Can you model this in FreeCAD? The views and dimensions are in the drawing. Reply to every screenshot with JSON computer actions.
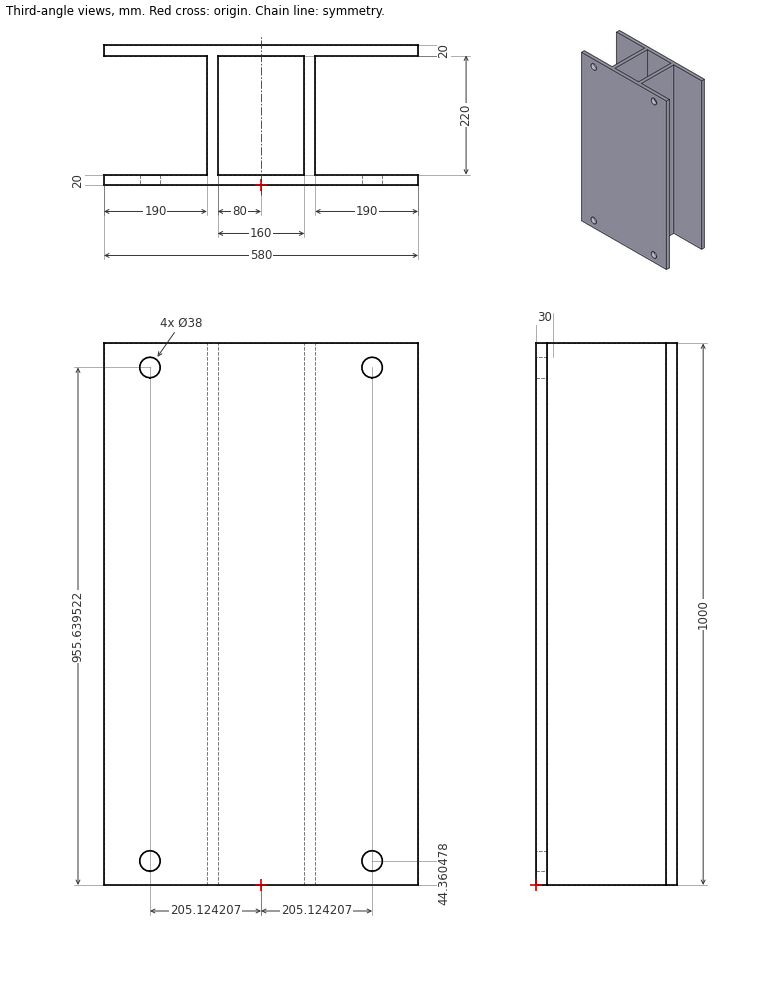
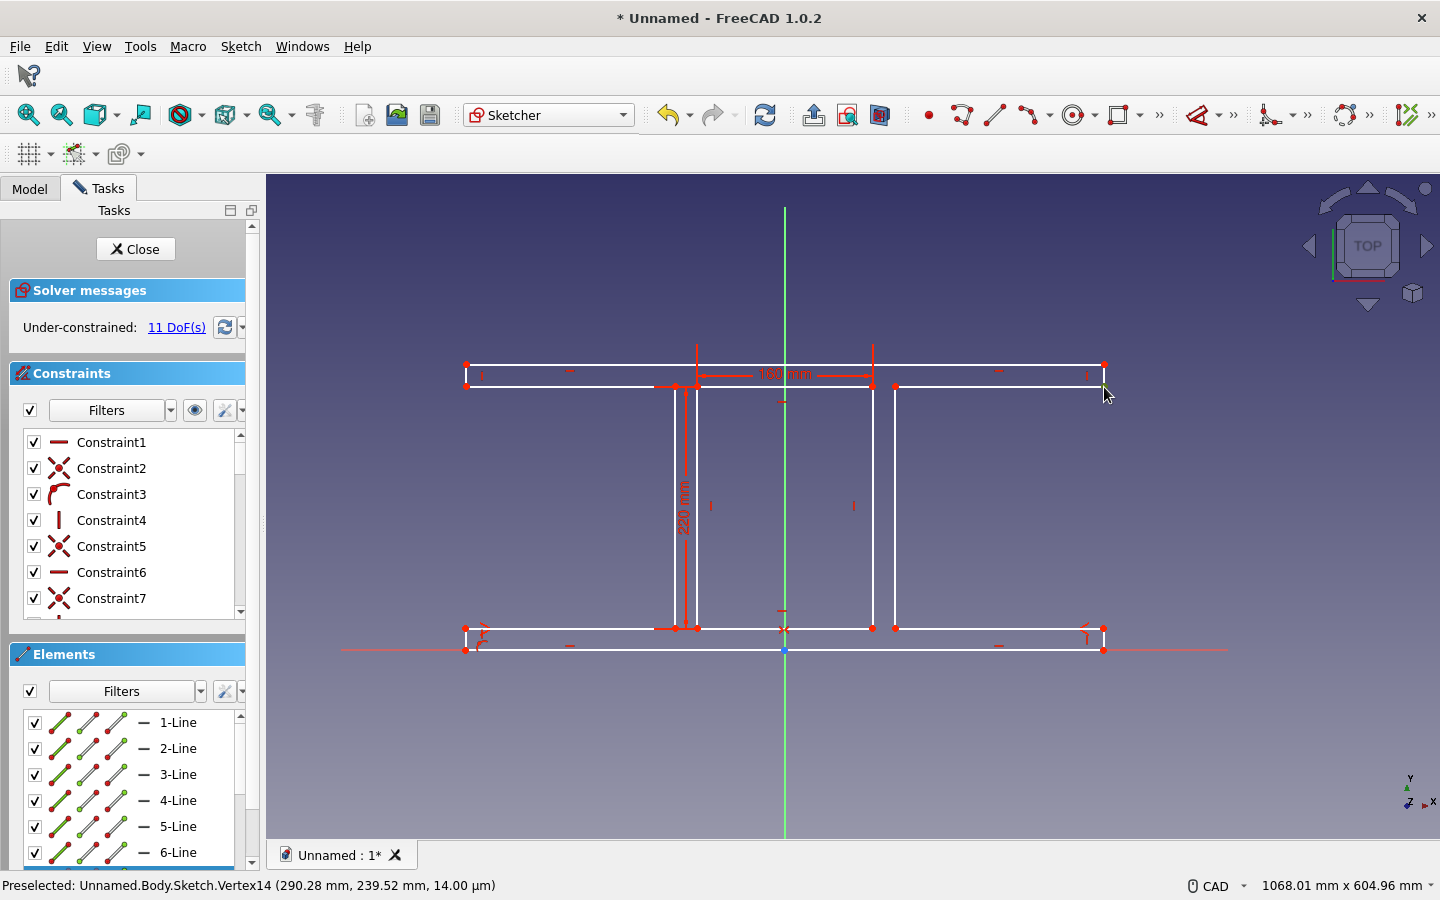
{"action": "left_click", "coordinate": [466, 387]}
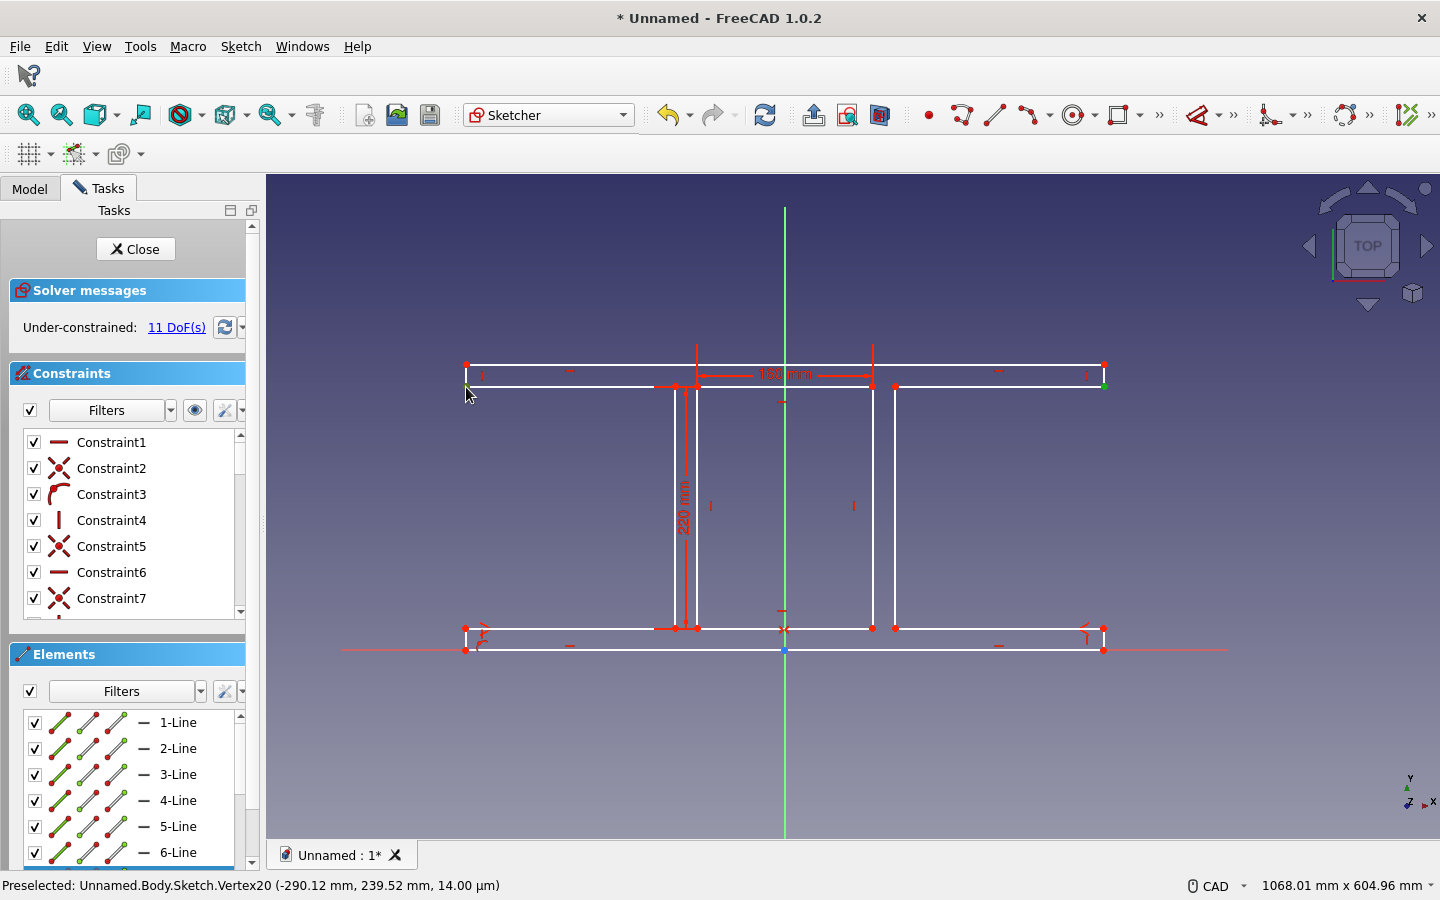
{"action": "left_click", "coordinate": [785, 768]}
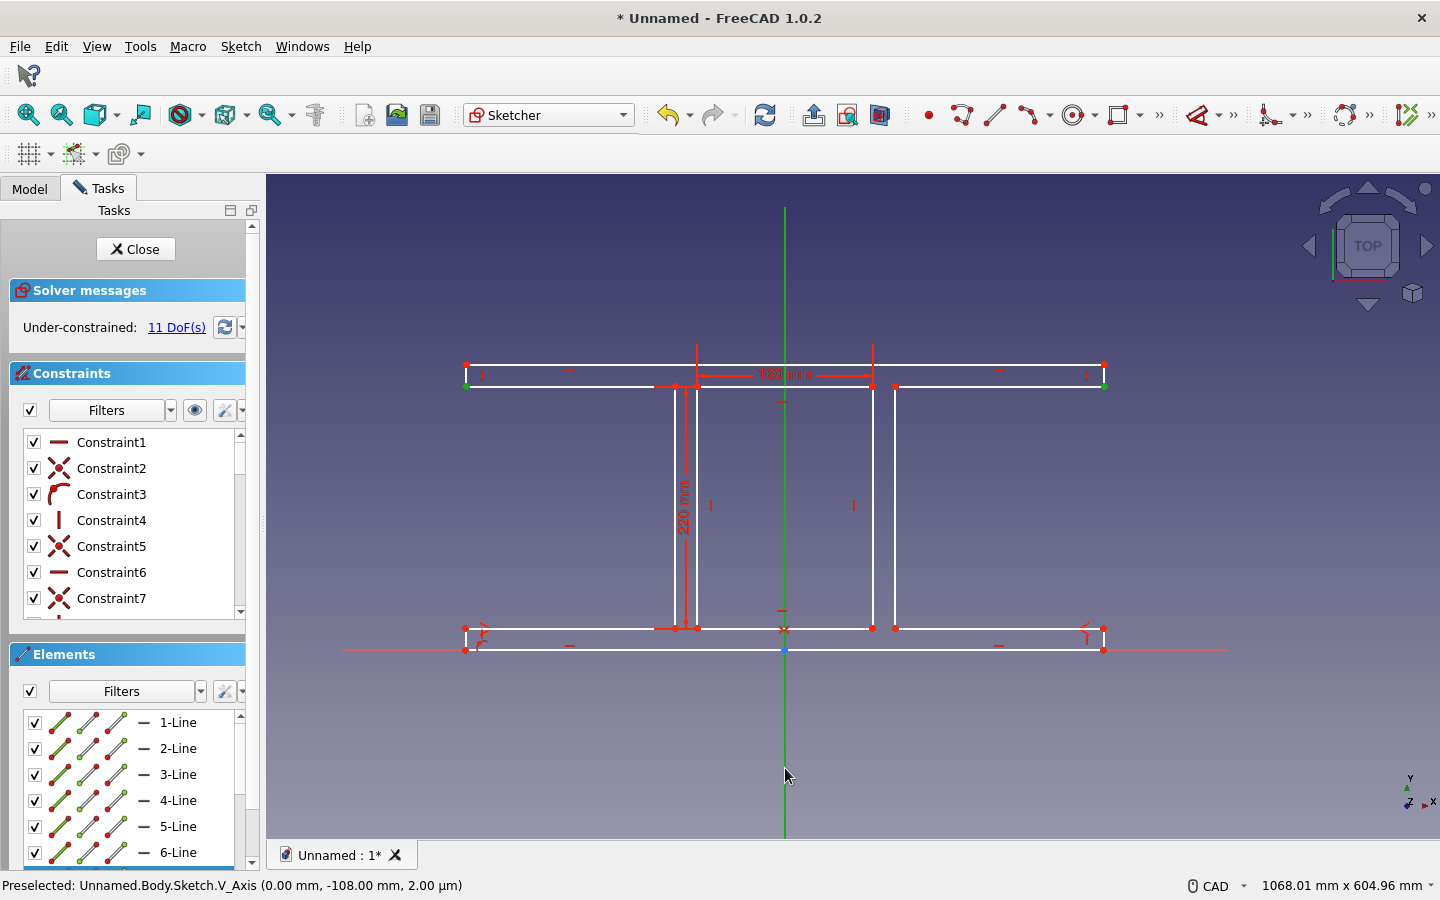
{"action": "key", "text": "s"}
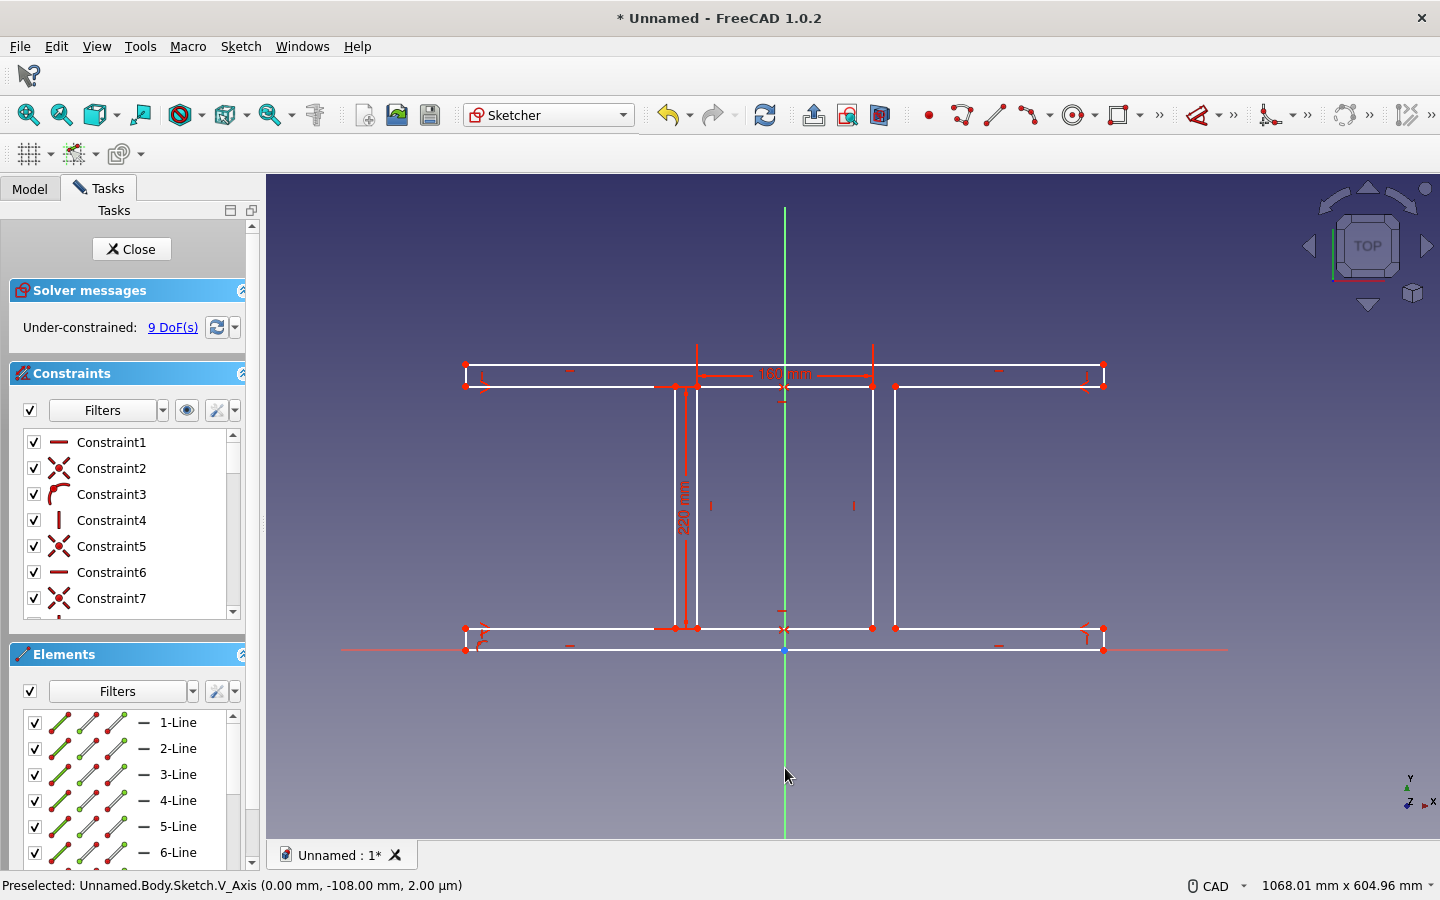
{"action": "key", "text": "d"}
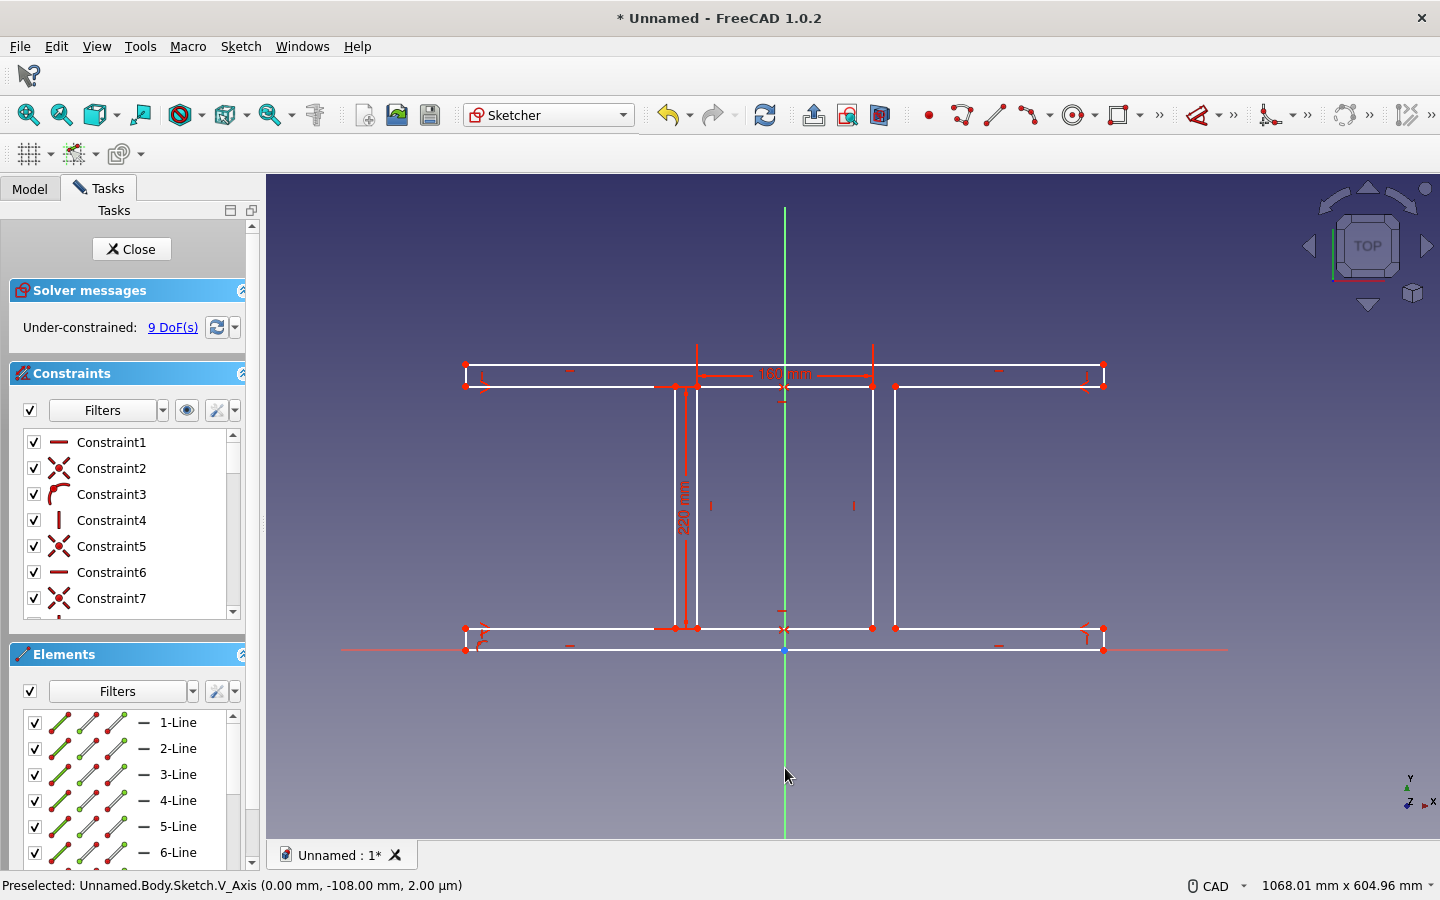
{"action": "scroll", "coordinate": [466, 640], "scroll_direction": "up", "scroll_amount": 3}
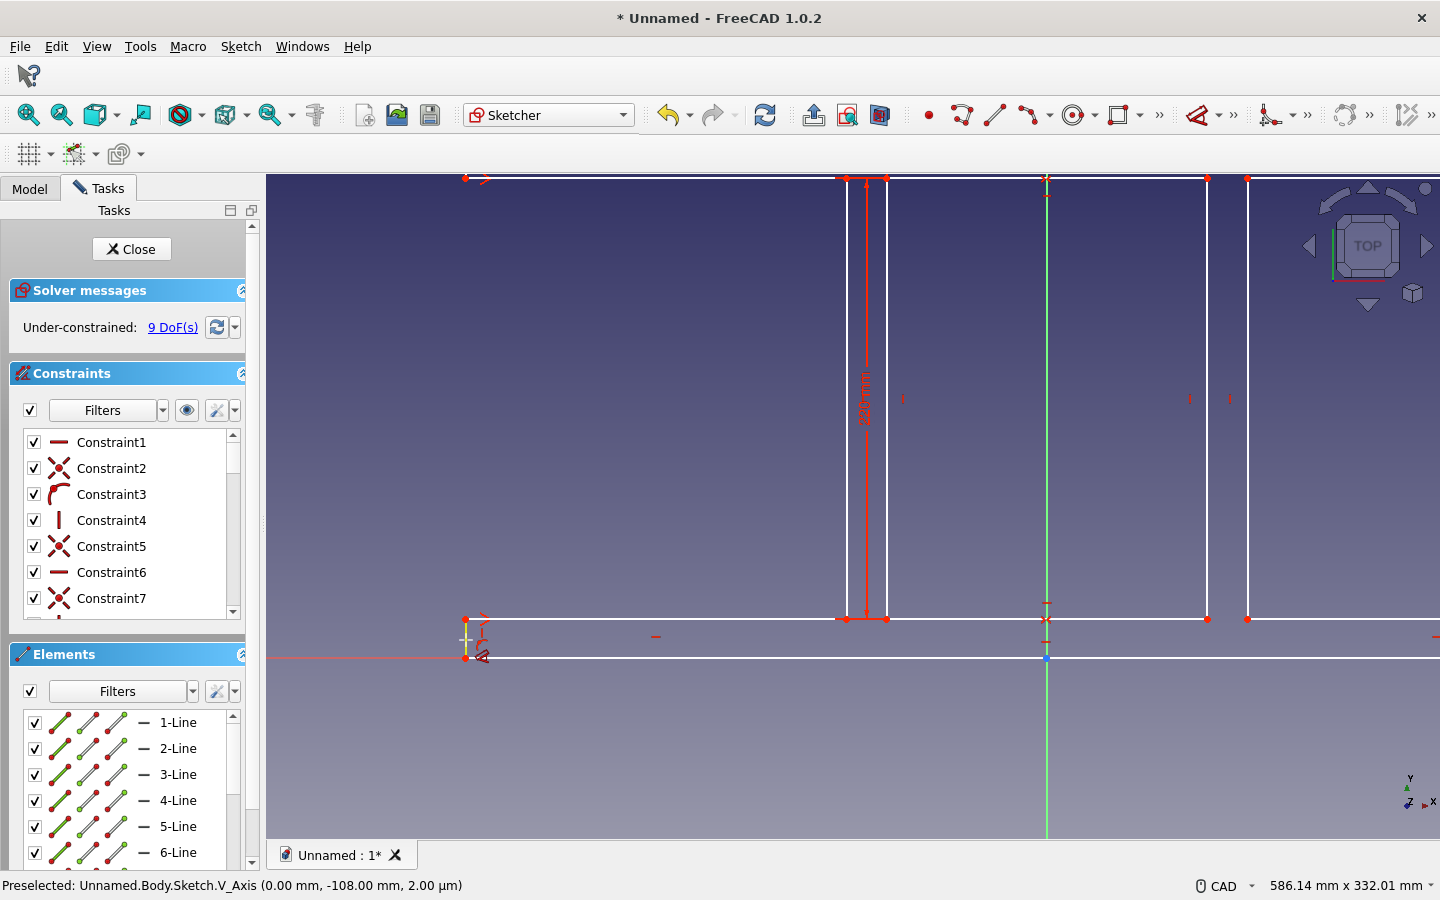
{"action": "left_click", "coordinate": [466, 639]}
{"action": "left_click", "coordinate": [432, 639]}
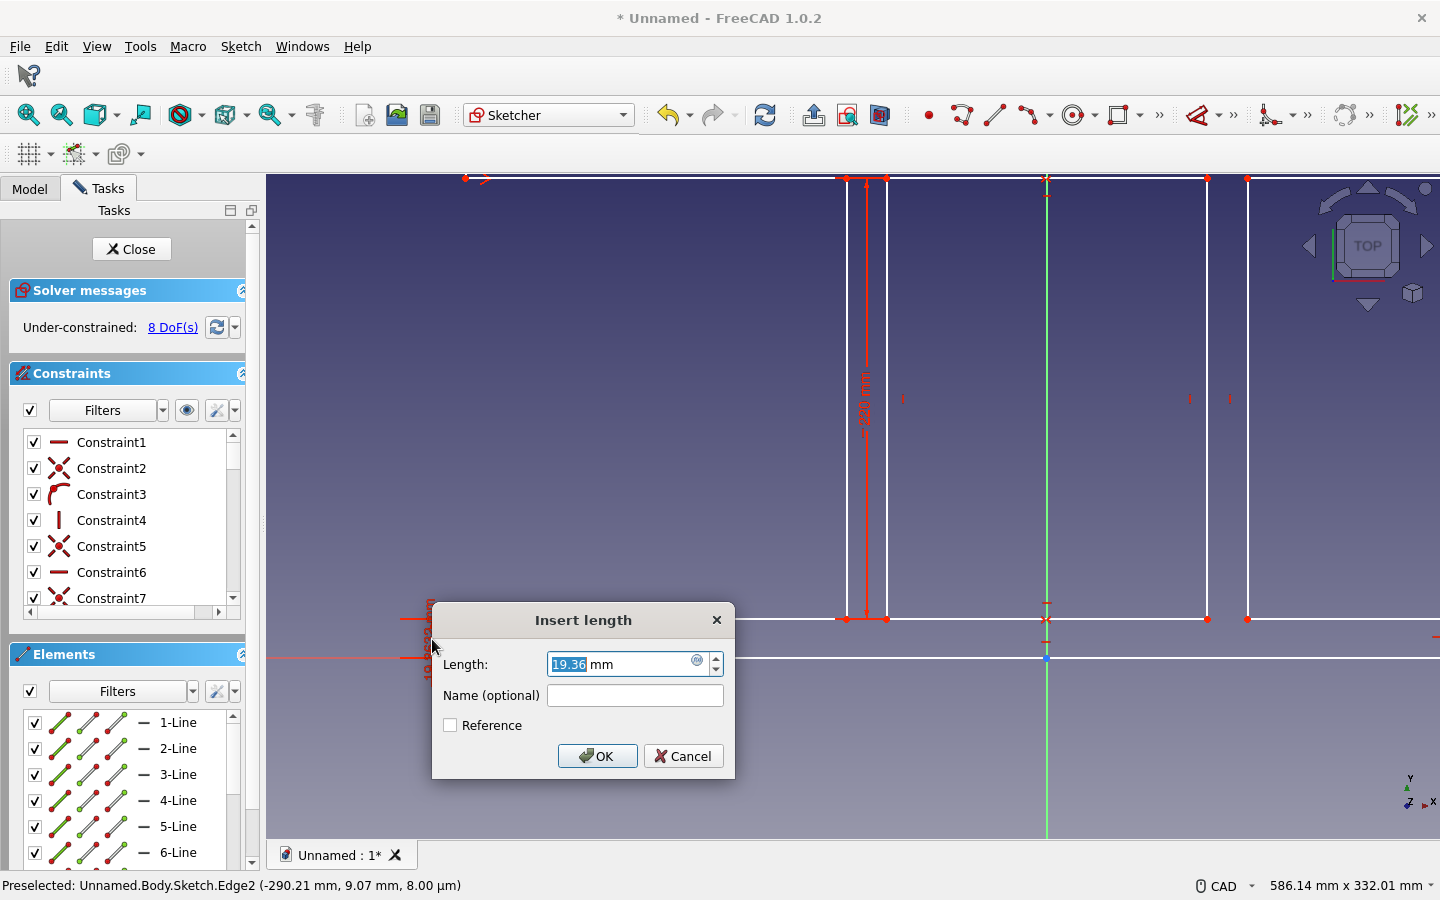
{"action": "type", "text": "20"}
{"action": "key", "text": "Return"}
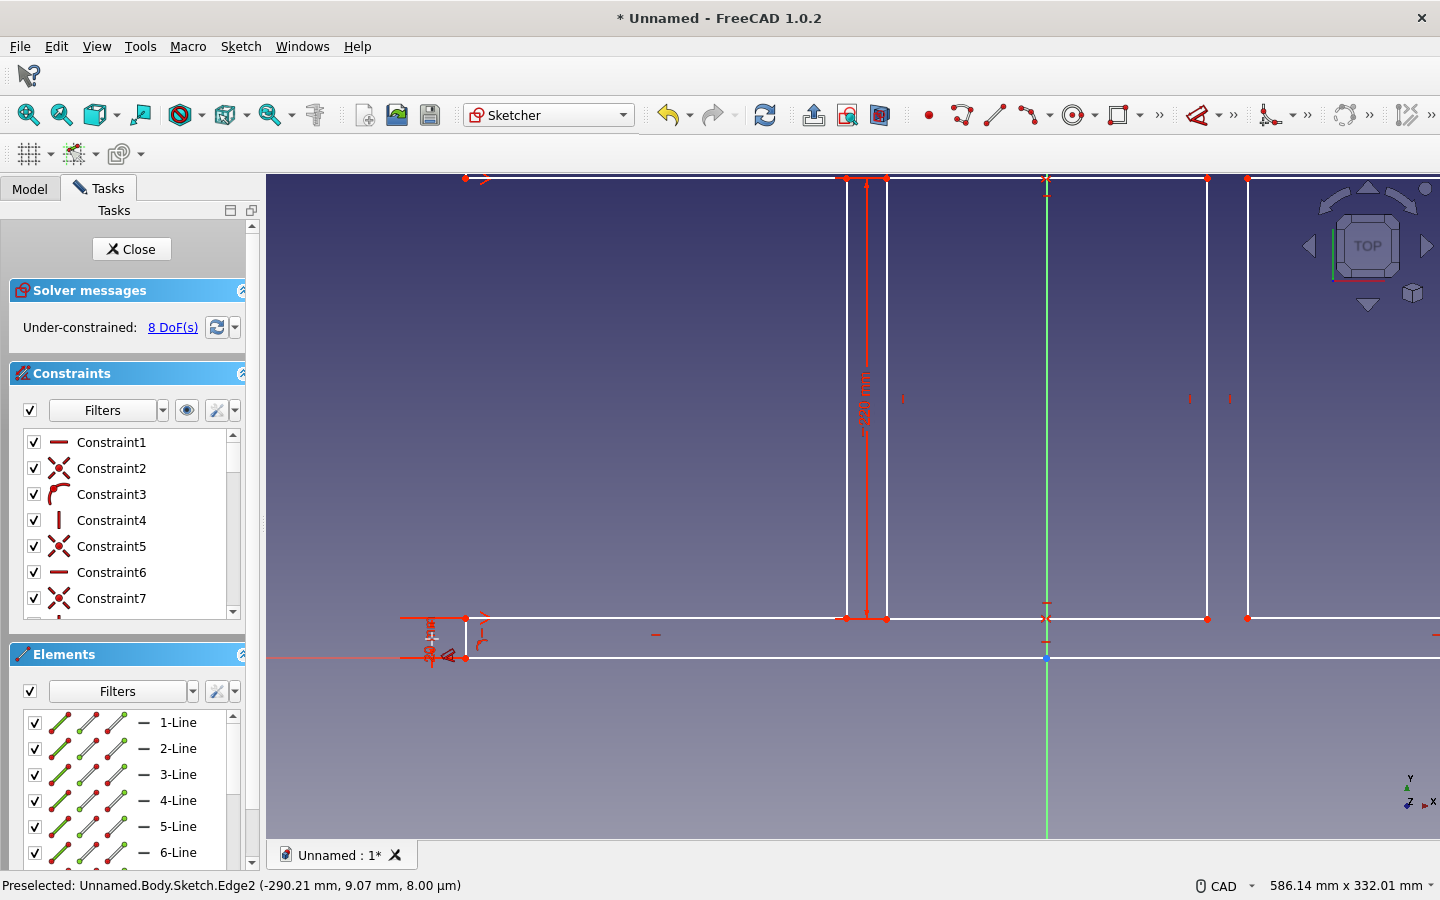
{"action": "scroll", "coordinate": [465, 639], "scroll_direction": "down", "scroll_amount": 3}